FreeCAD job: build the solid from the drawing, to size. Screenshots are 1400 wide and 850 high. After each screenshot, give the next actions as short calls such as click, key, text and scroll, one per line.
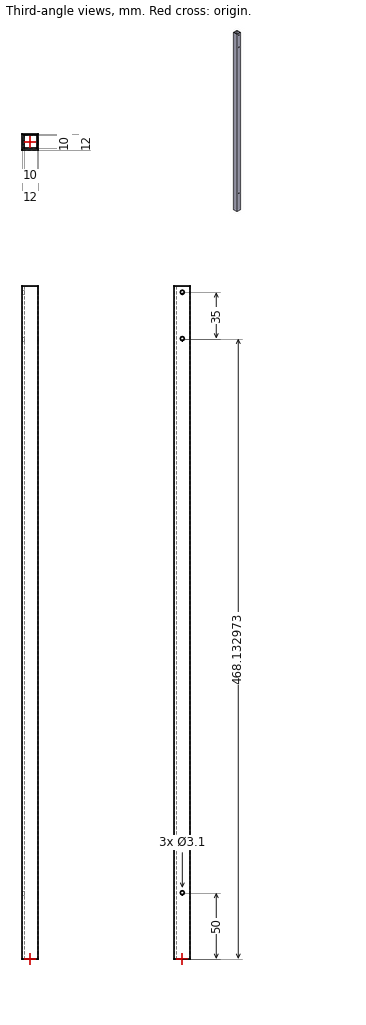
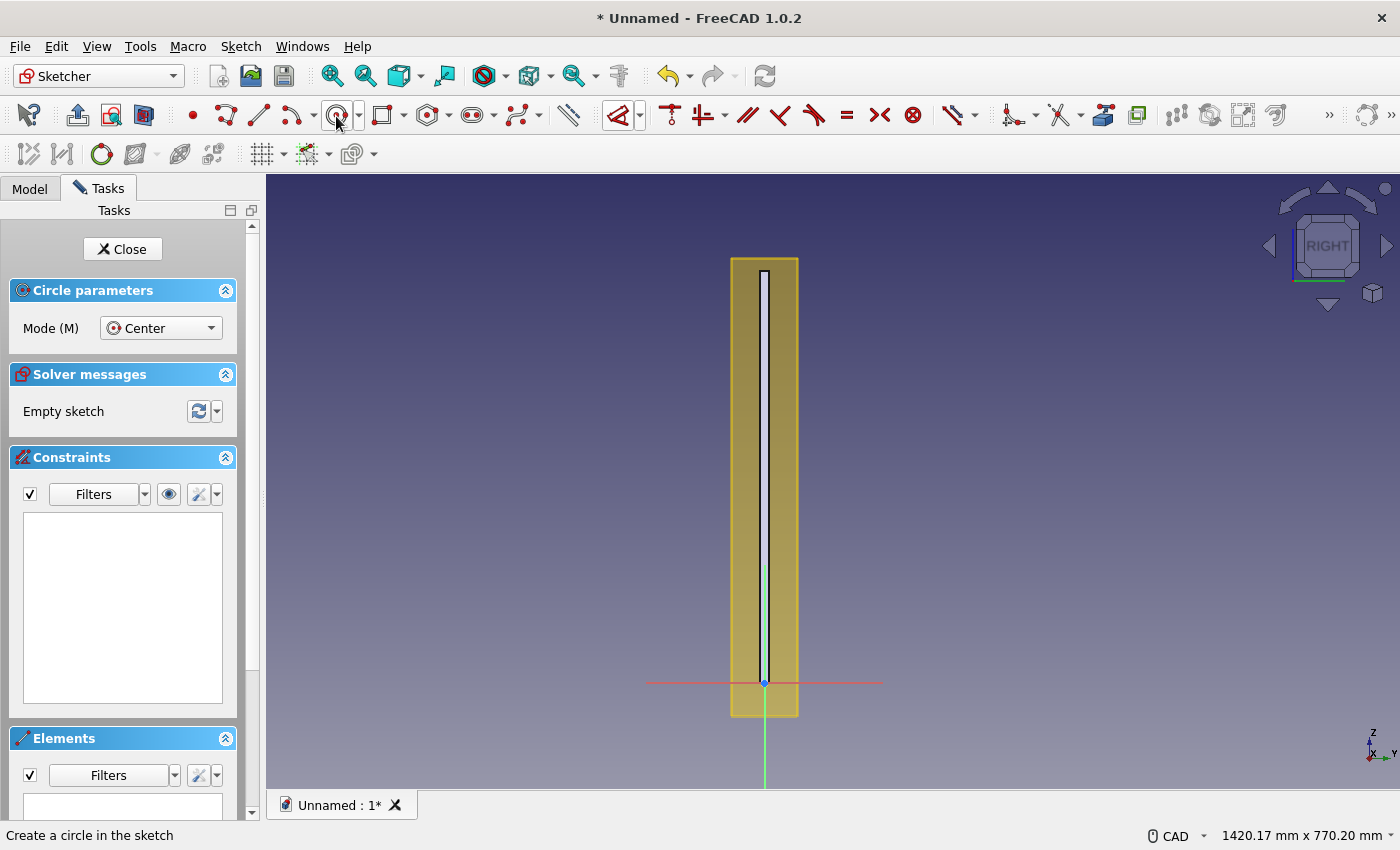
scroll(765, 643, up, 15)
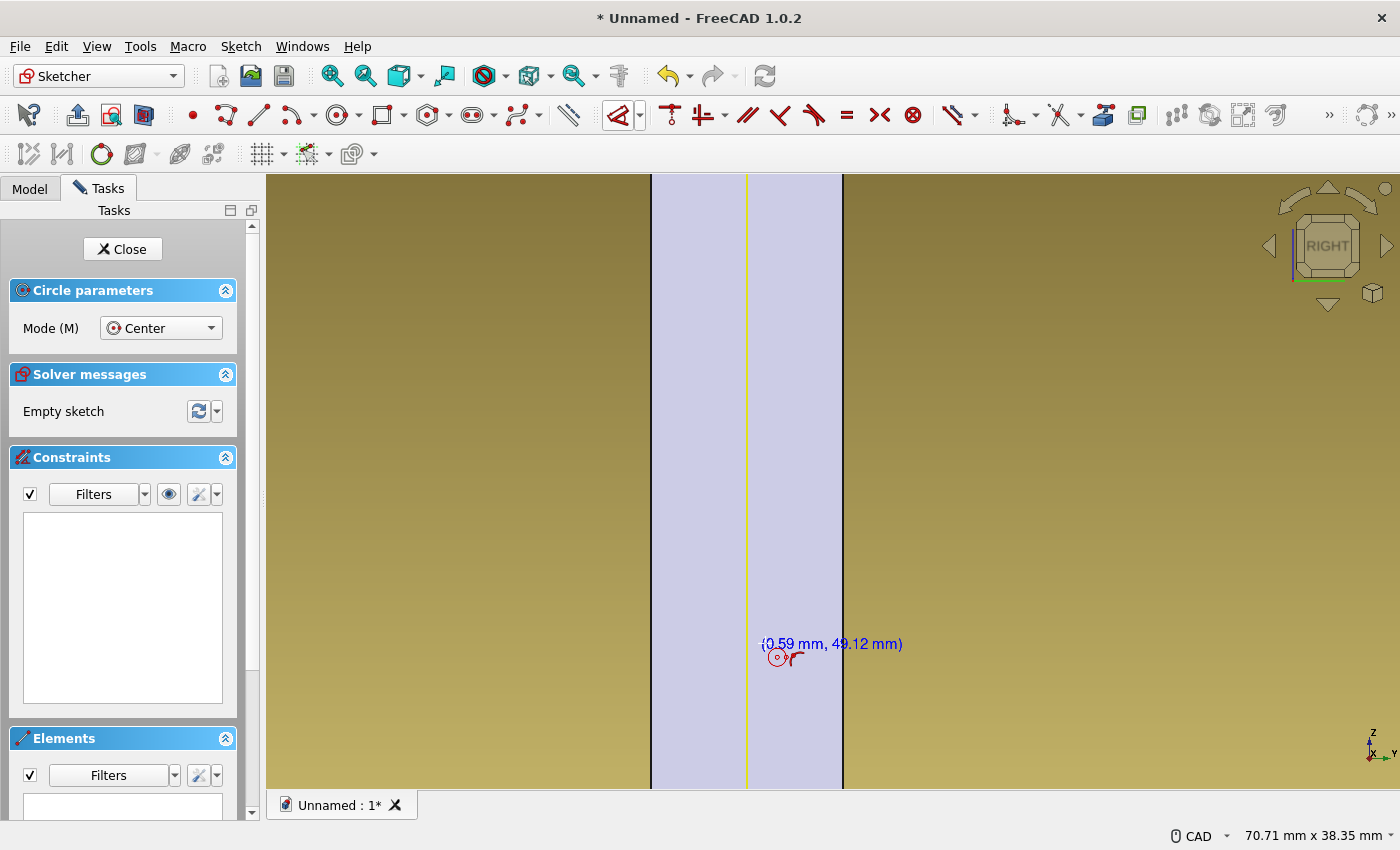
scroll(765, 644, down, 15)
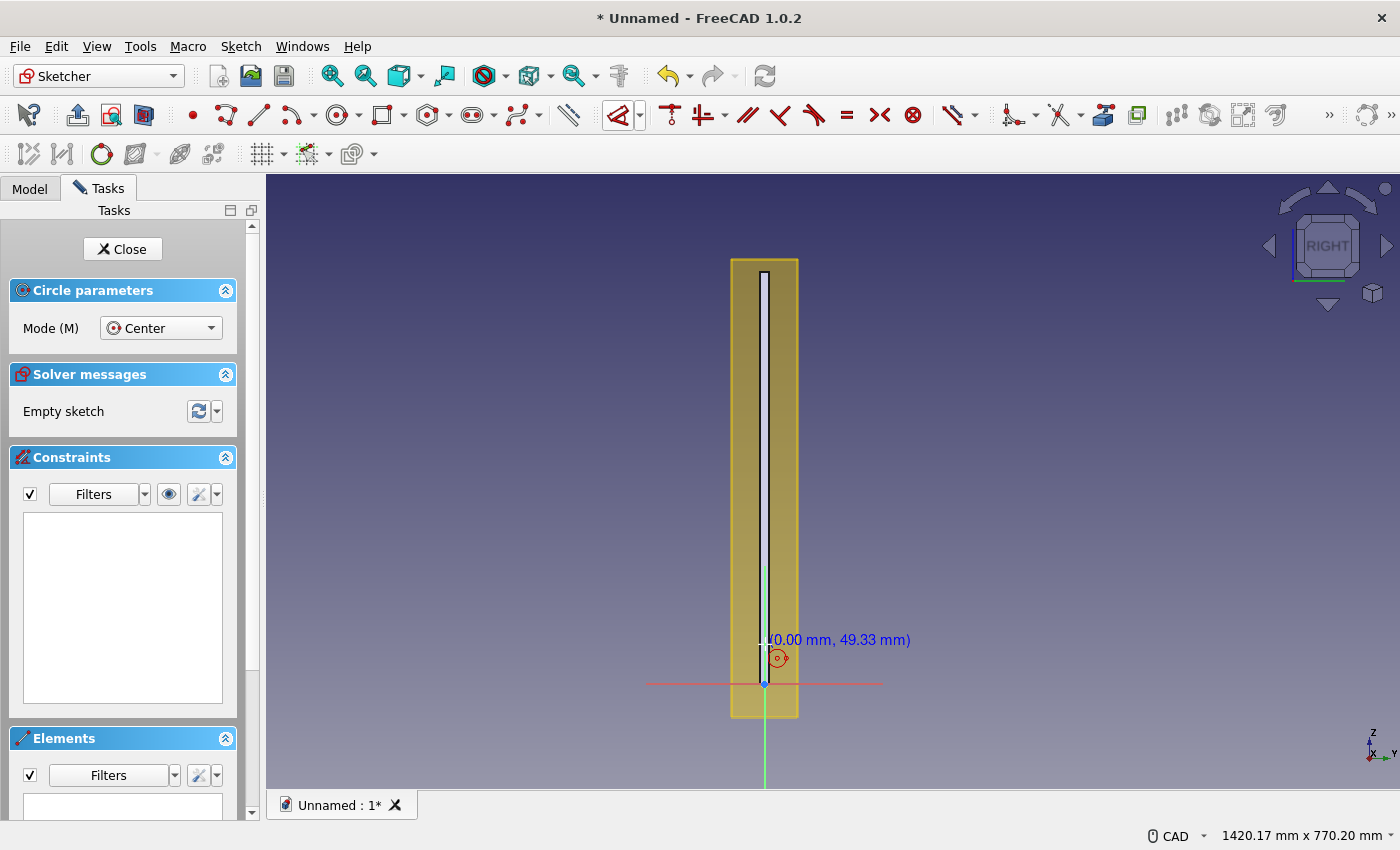
click(765, 644)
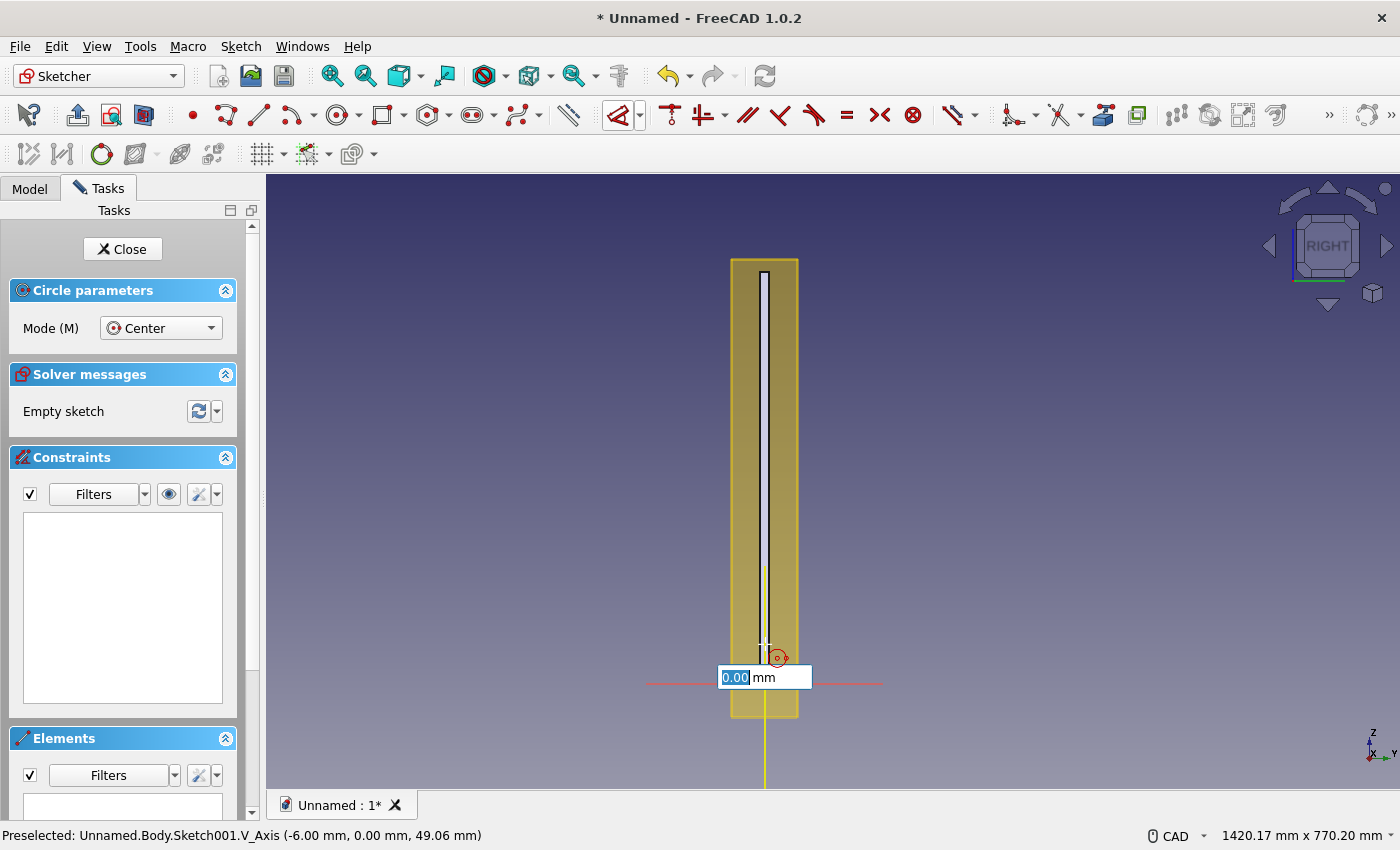
scroll(766, 644, up, 14)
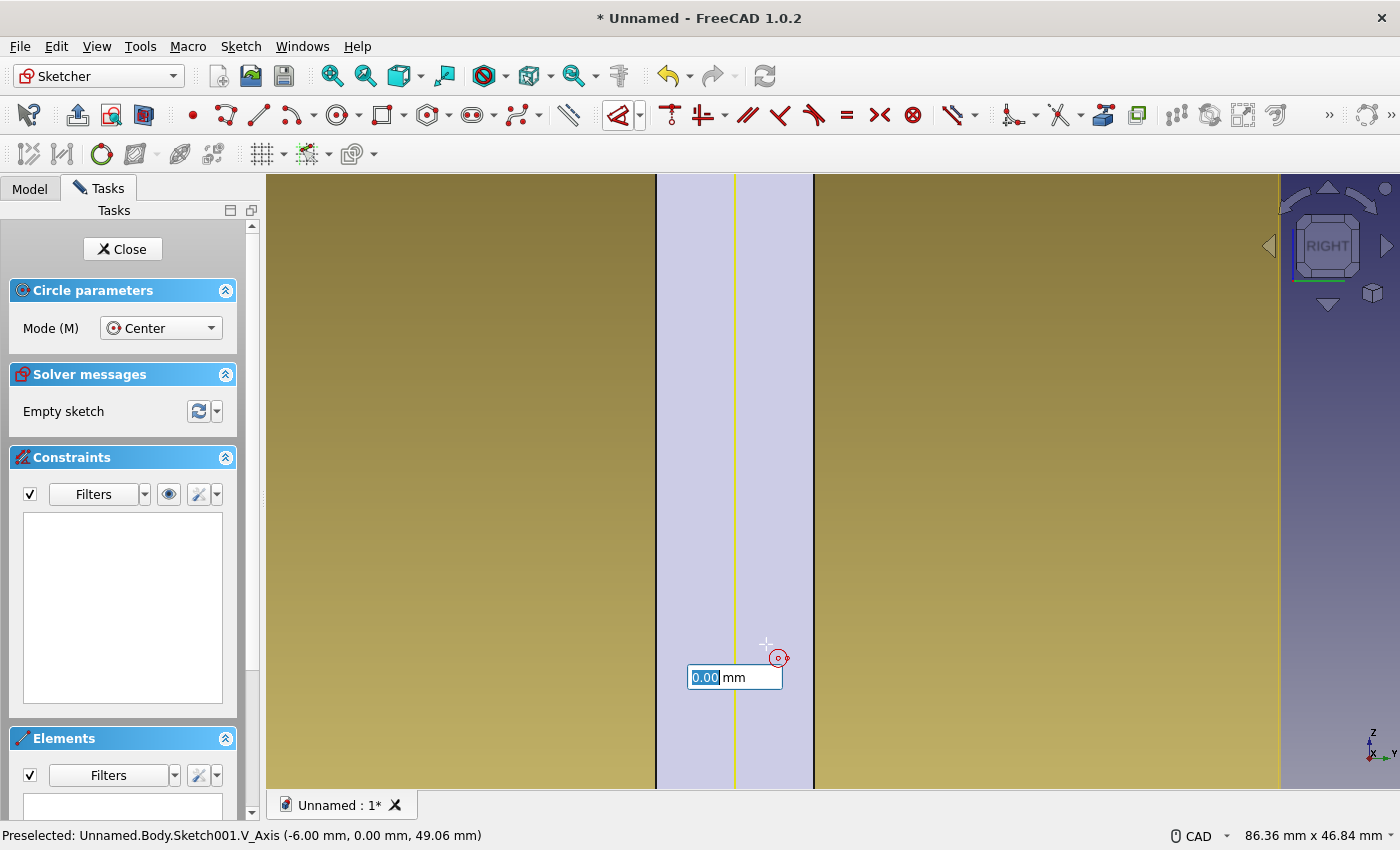
click(754, 629)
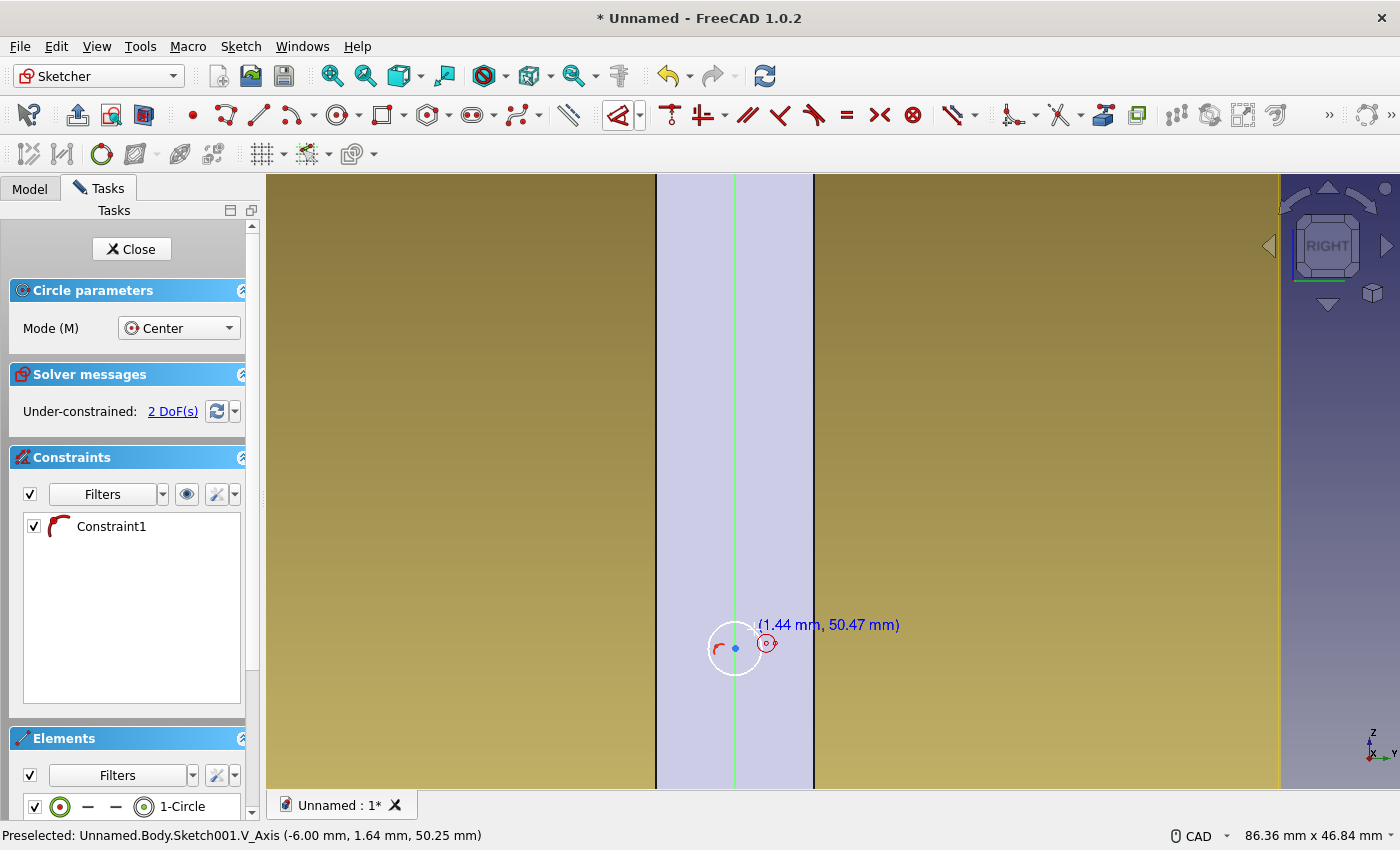
scroll(766, 644, down, 14)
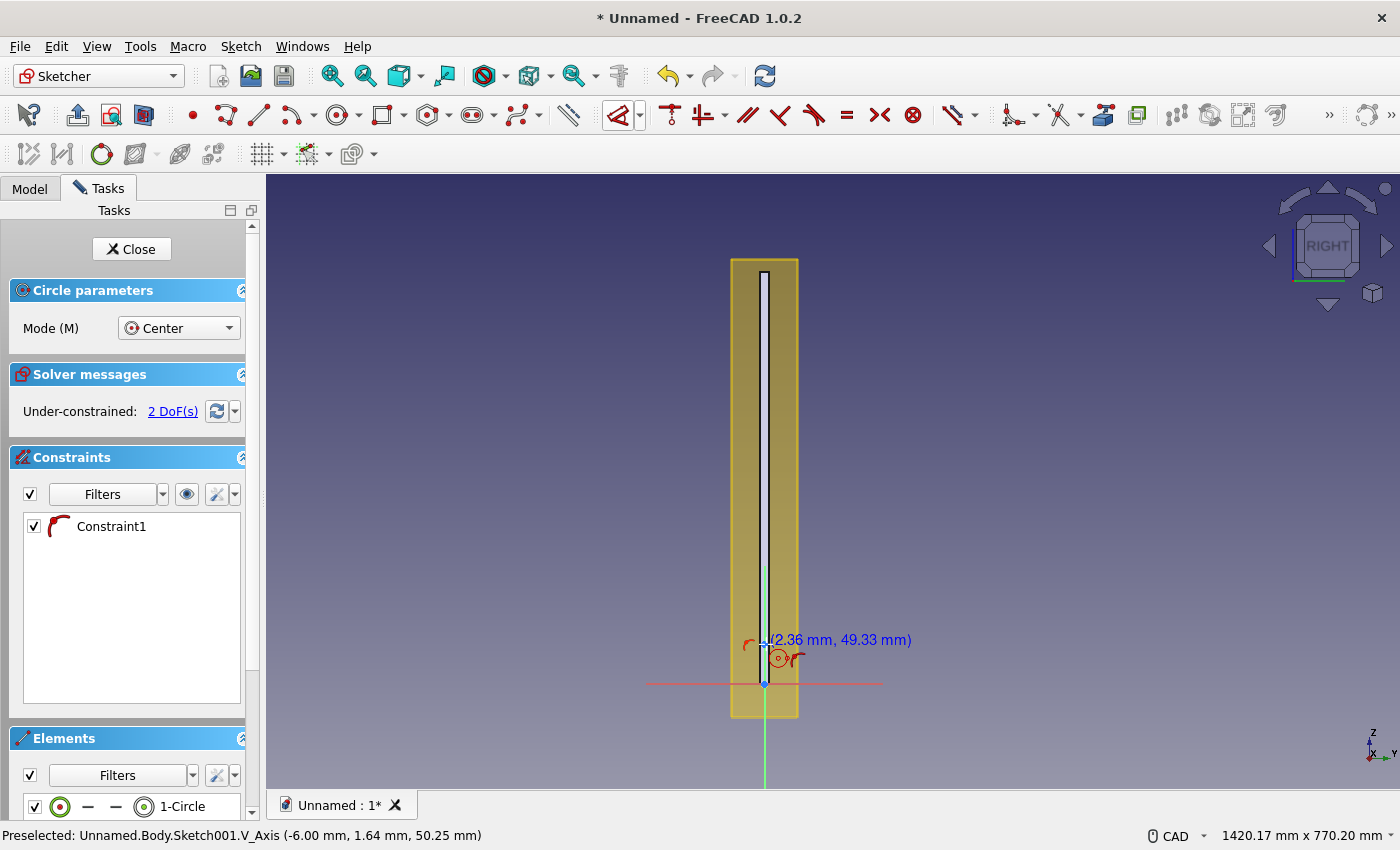
scroll(765, 310, up, 15)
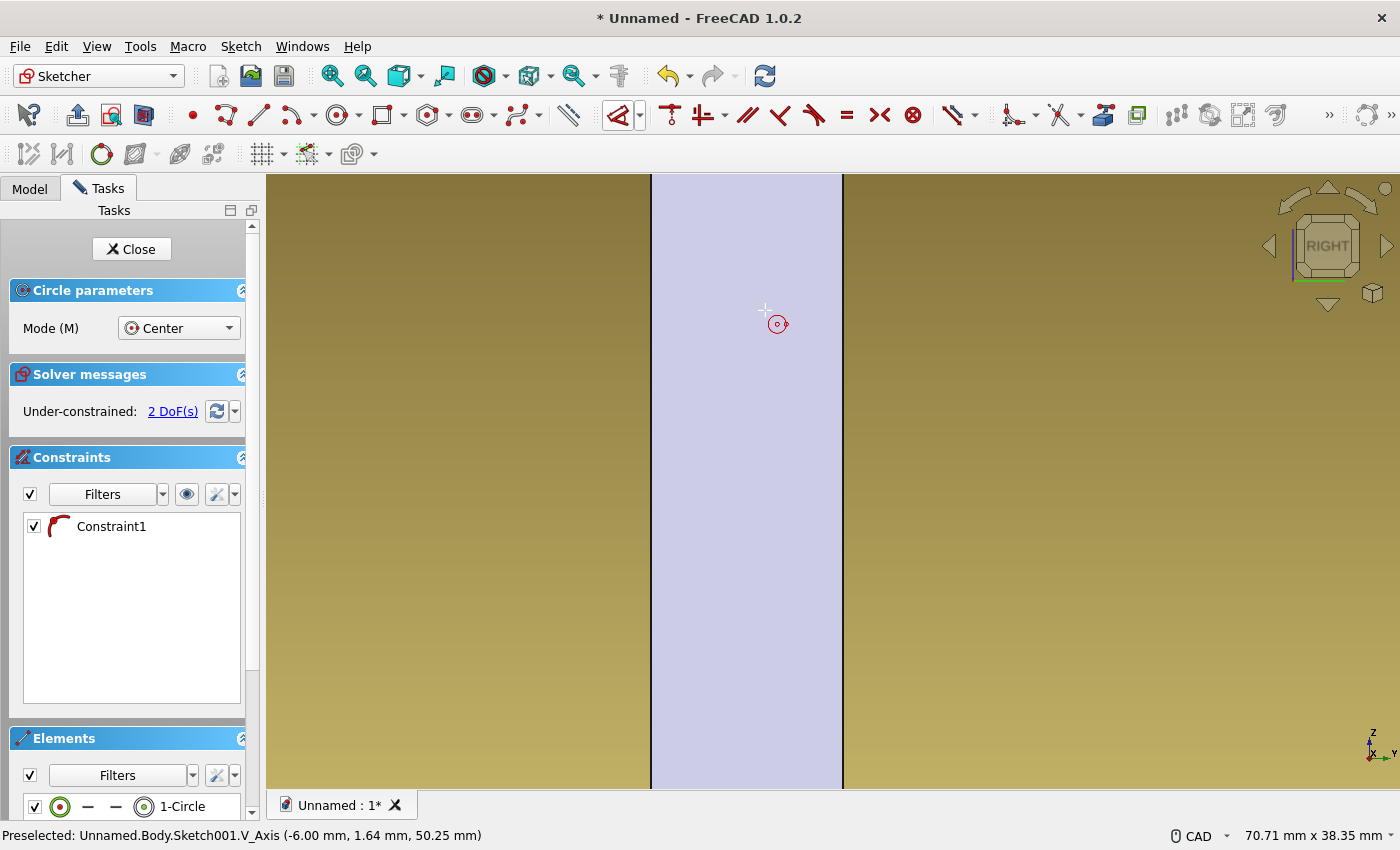
scroll(765, 309, down, 15)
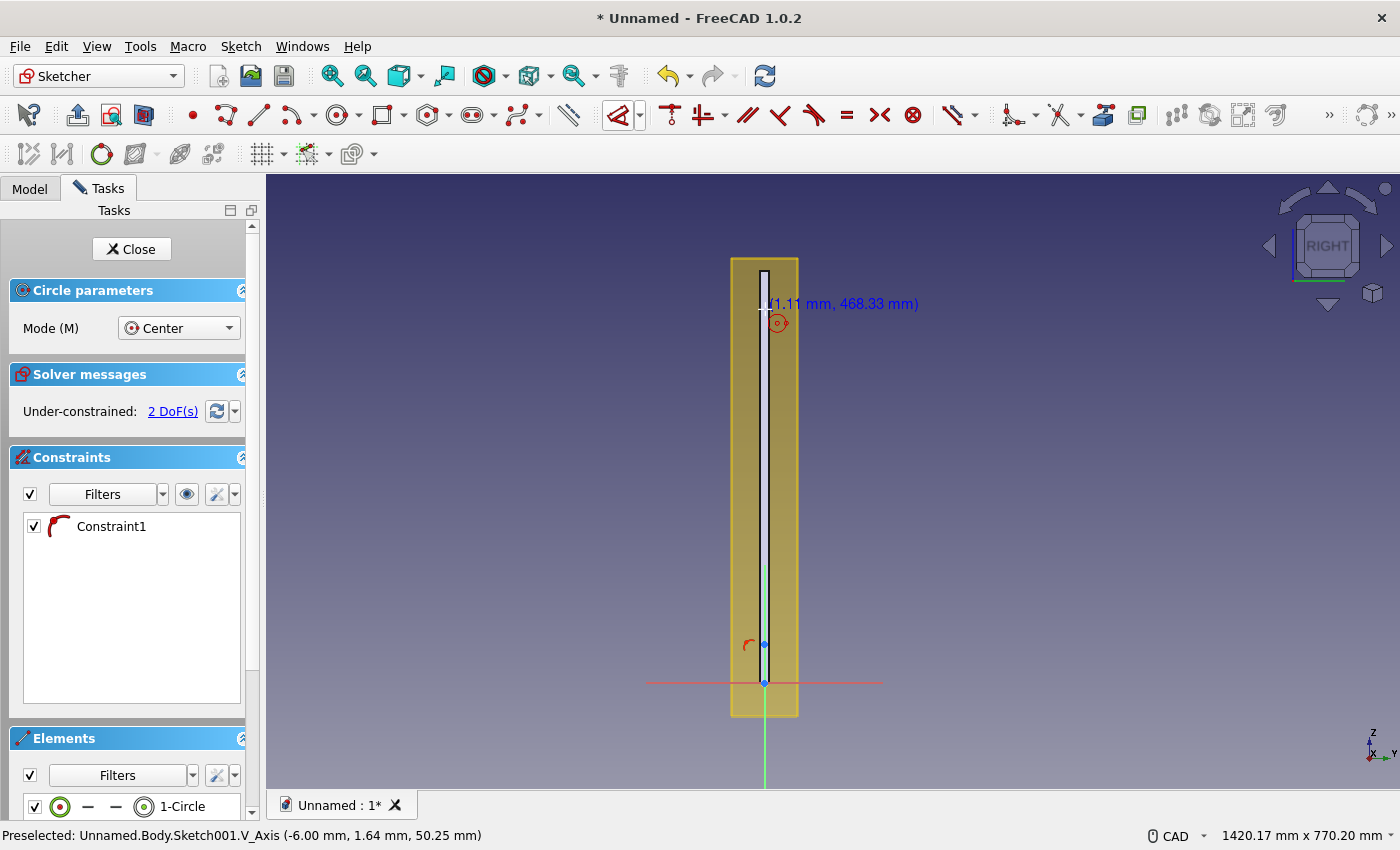
click(765, 309)